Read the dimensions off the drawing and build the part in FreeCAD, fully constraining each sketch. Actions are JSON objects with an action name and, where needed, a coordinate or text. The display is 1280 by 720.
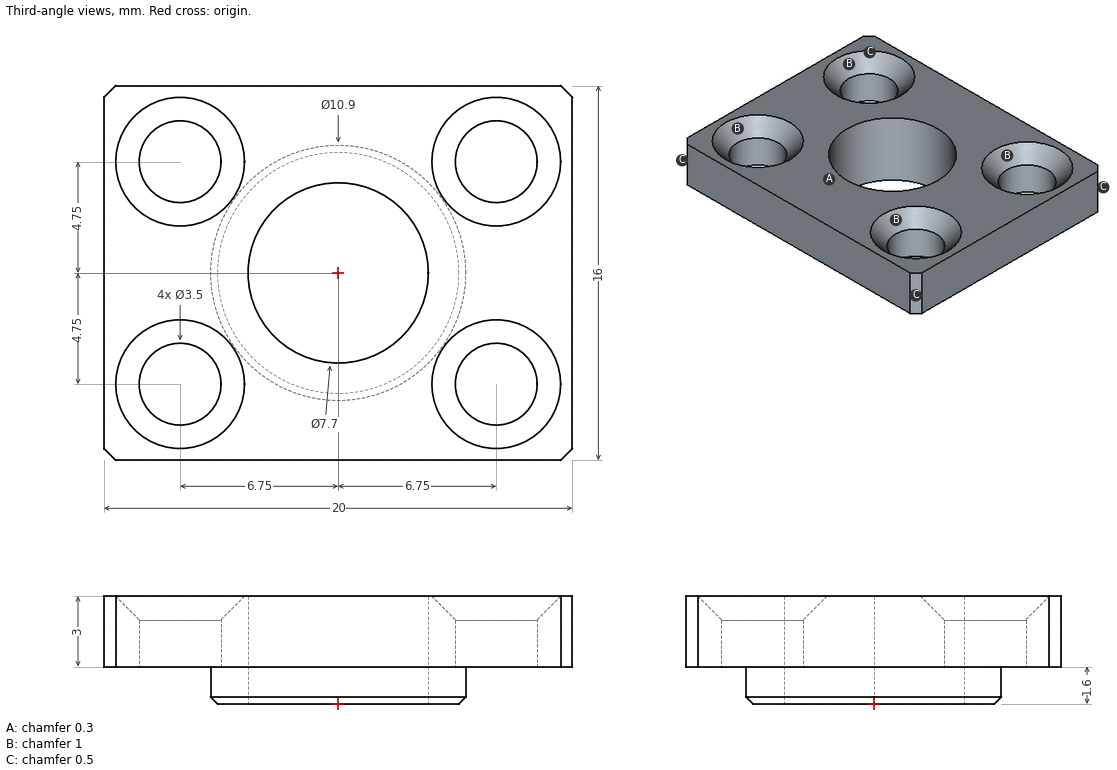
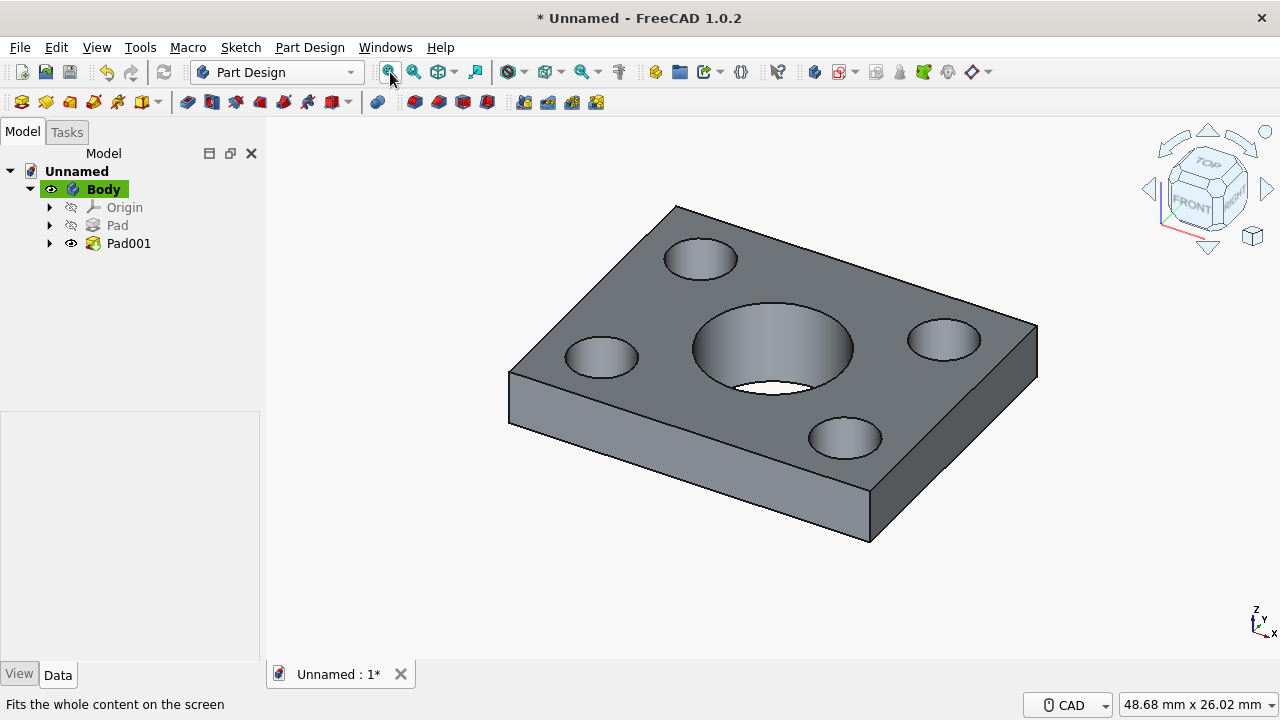
{"action": "key", "text": "0"}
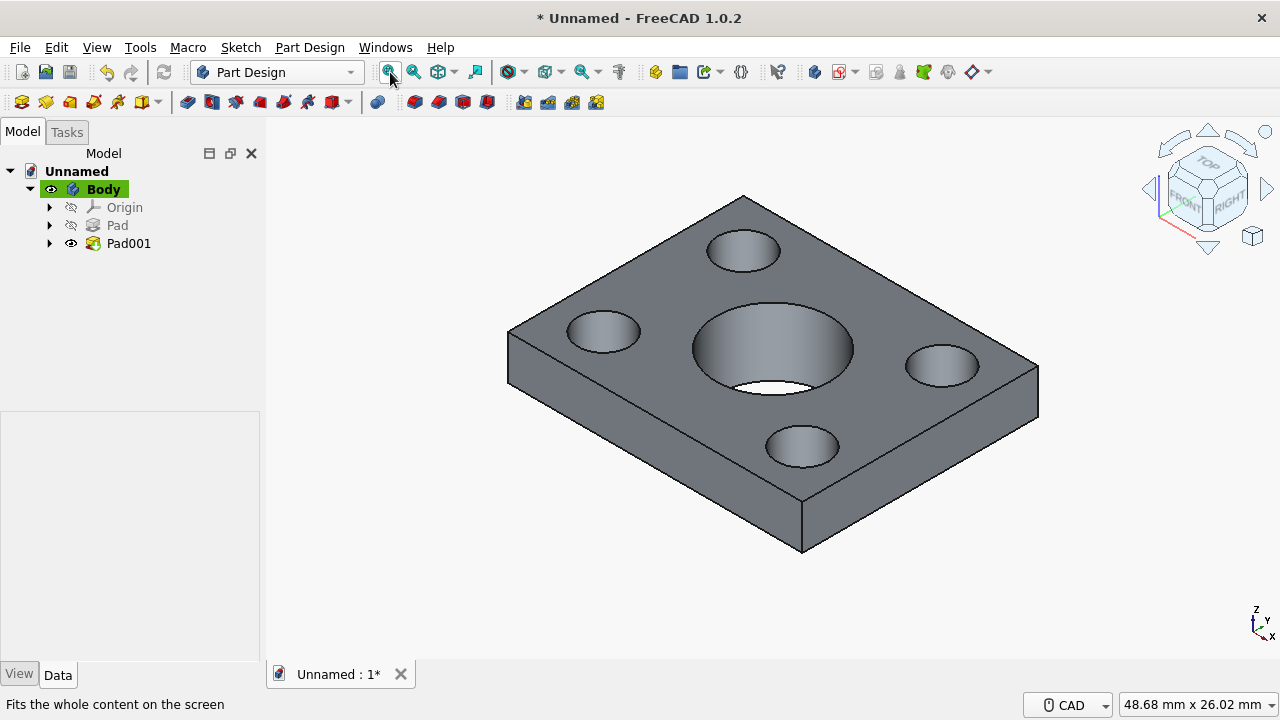
{"action": "key", "text": "2"}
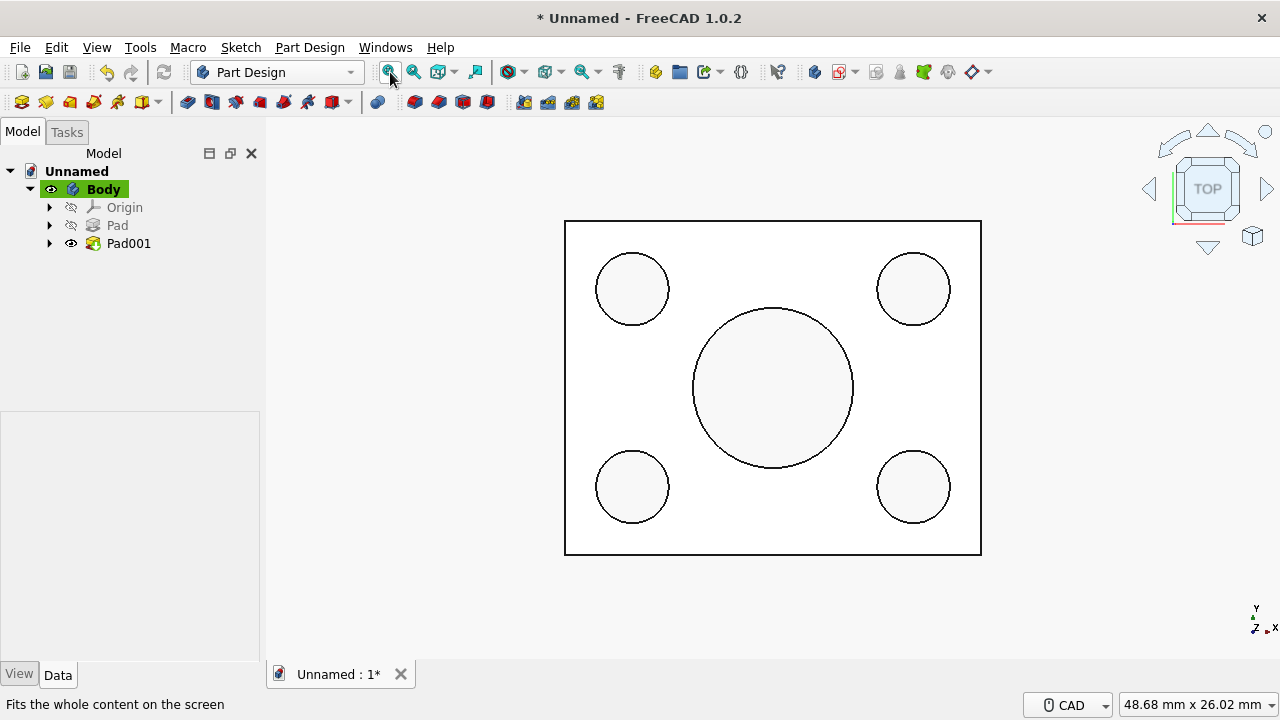
{"action": "key", "text": "1"}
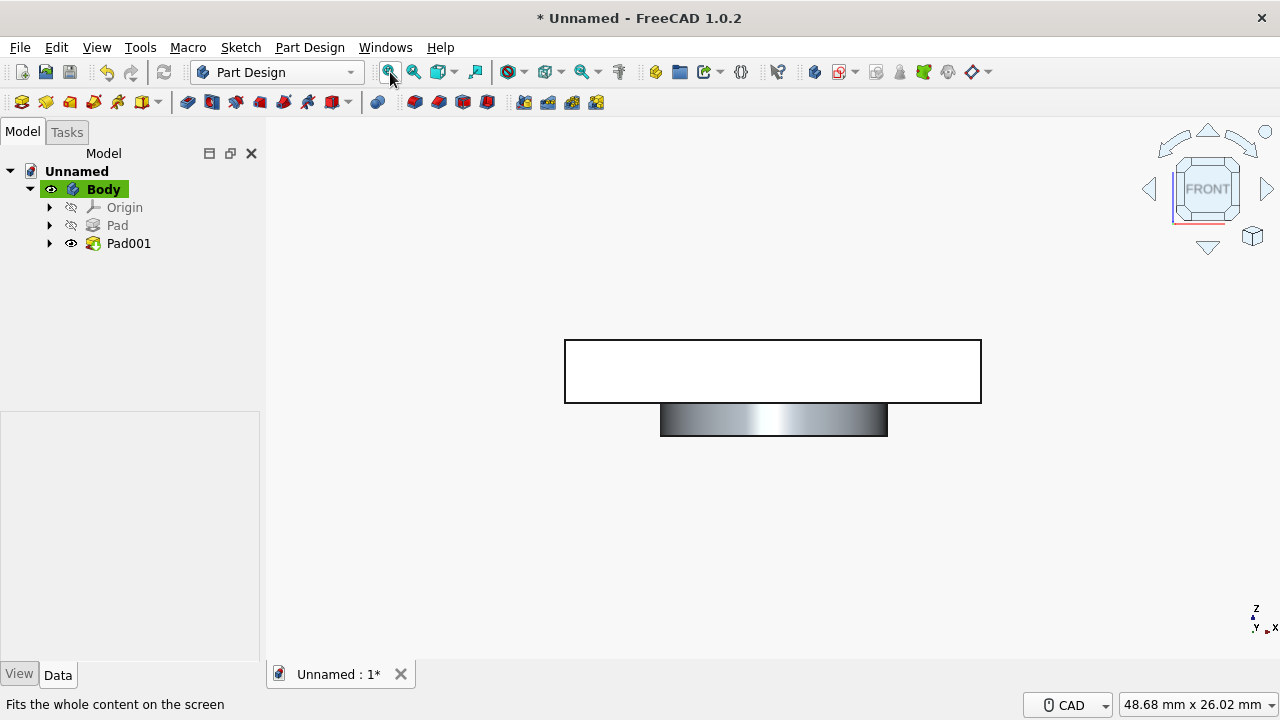
{"action": "key", "text": "v f"}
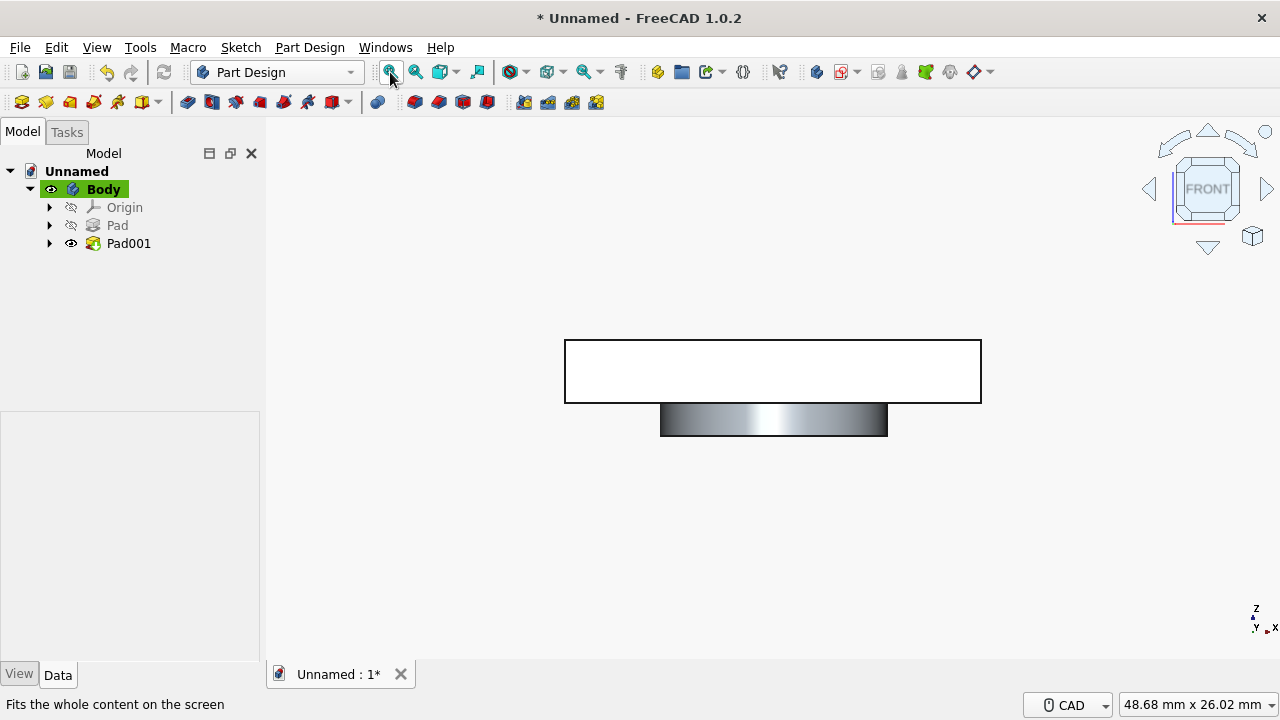
{"action": "left_click", "coordinate": [681, 435]}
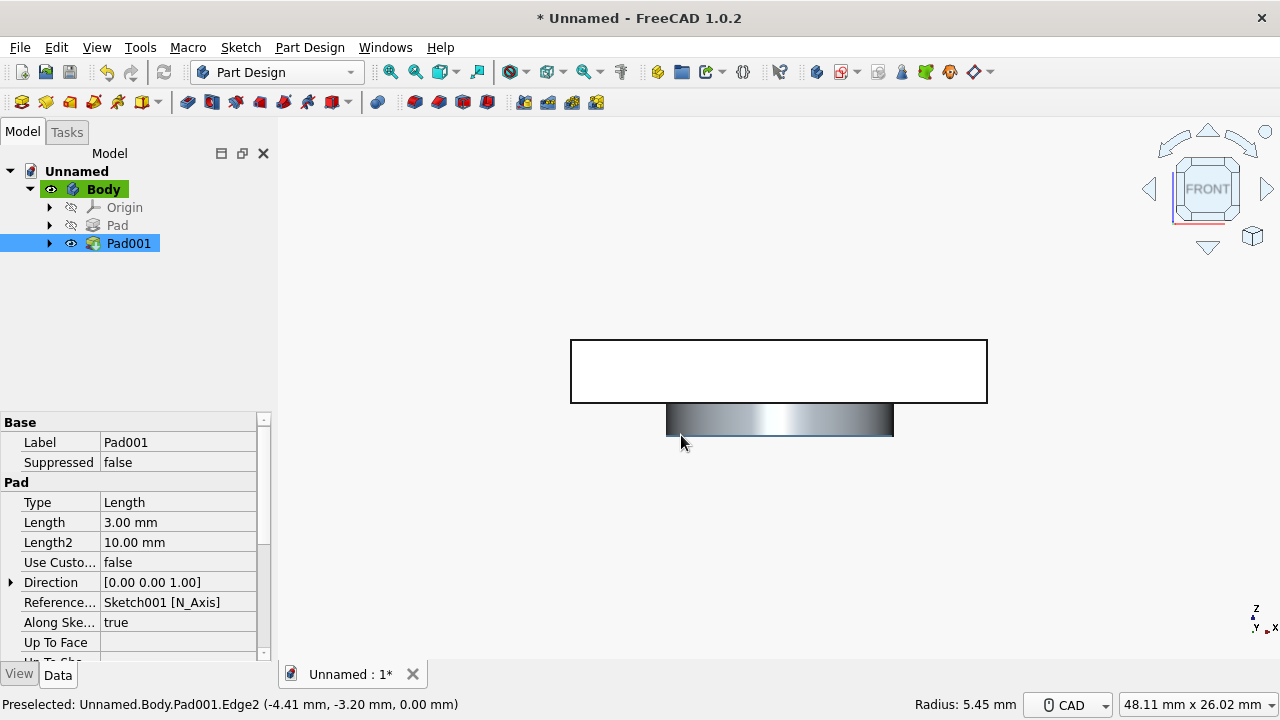
{"action": "left_click", "coordinate": [440, 102]}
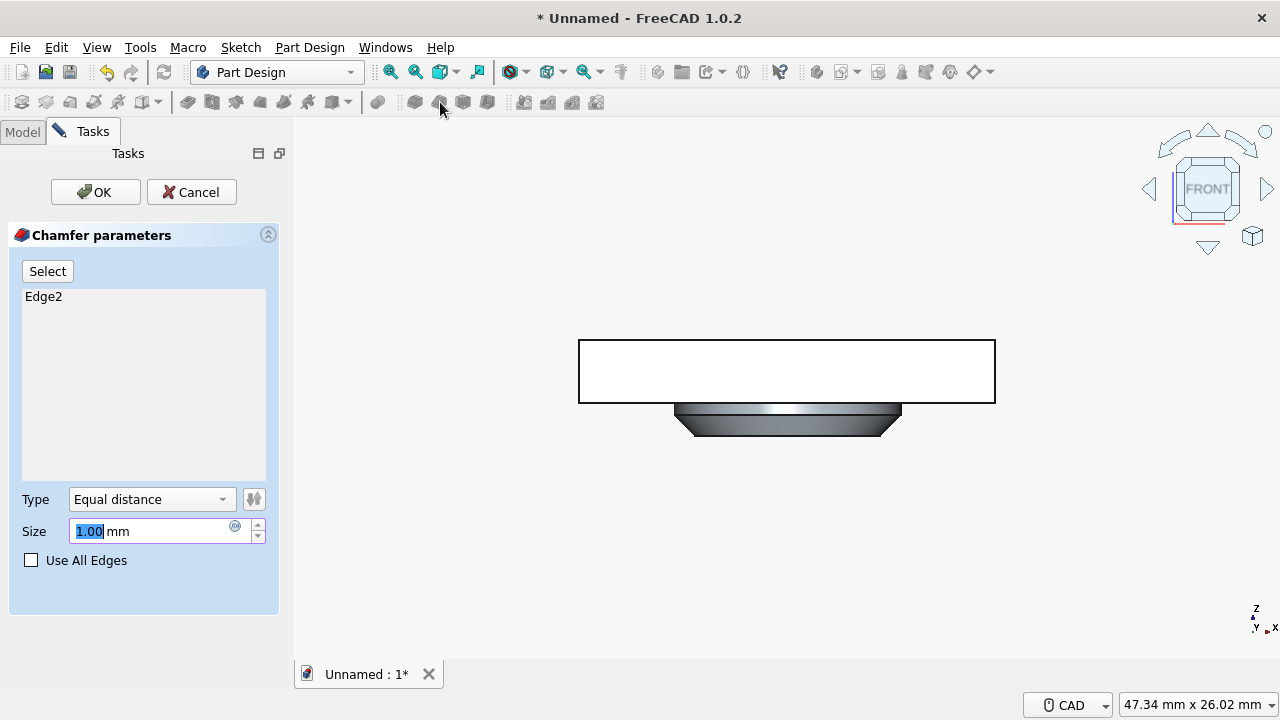
{"action": "type", "text": "0.3"}
{"action": "key", "text": "Tab"}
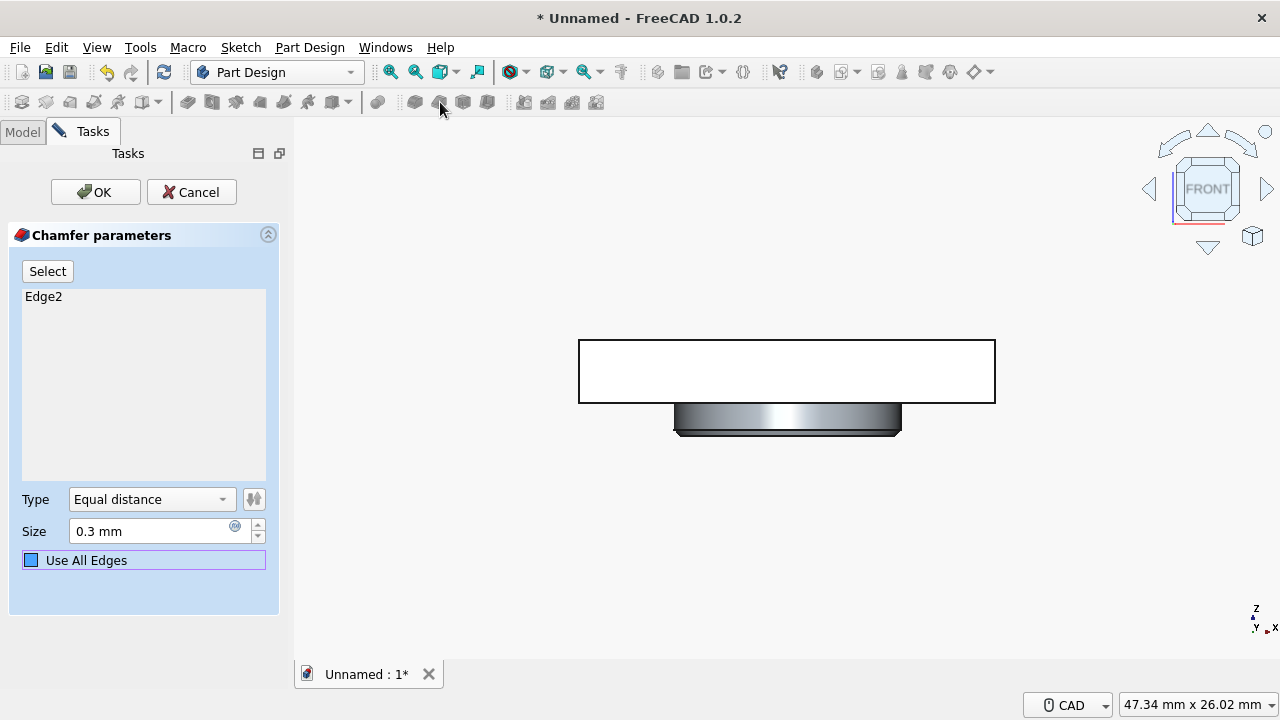
{"action": "left_click", "coordinate": [96, 192]}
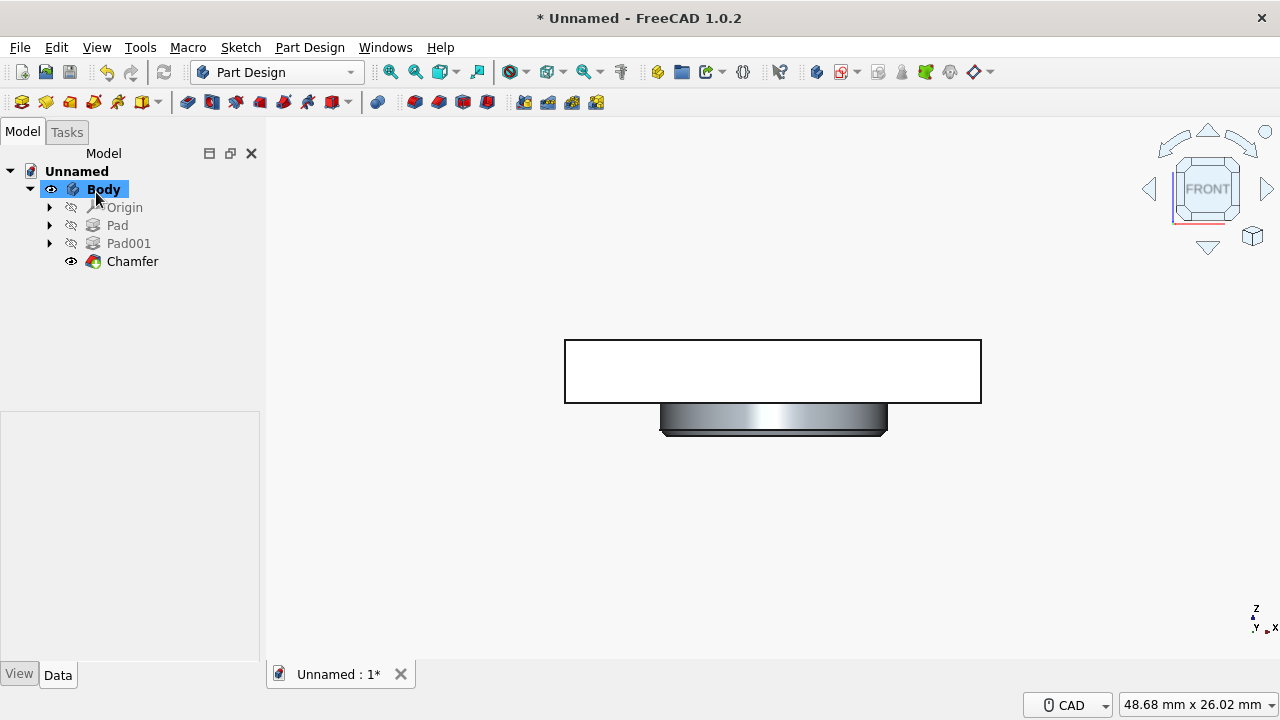
{"action": "left_click", "coordinate": [392, 72]}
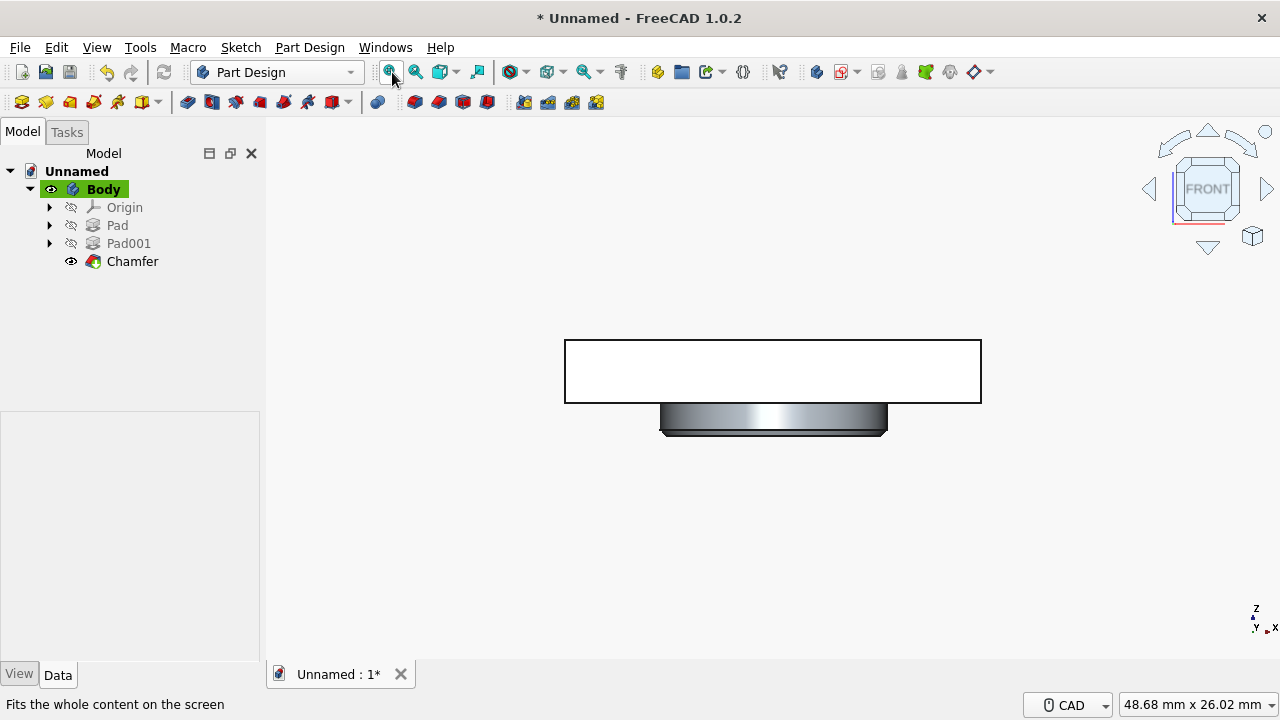
{"action": "key", "text": "0"}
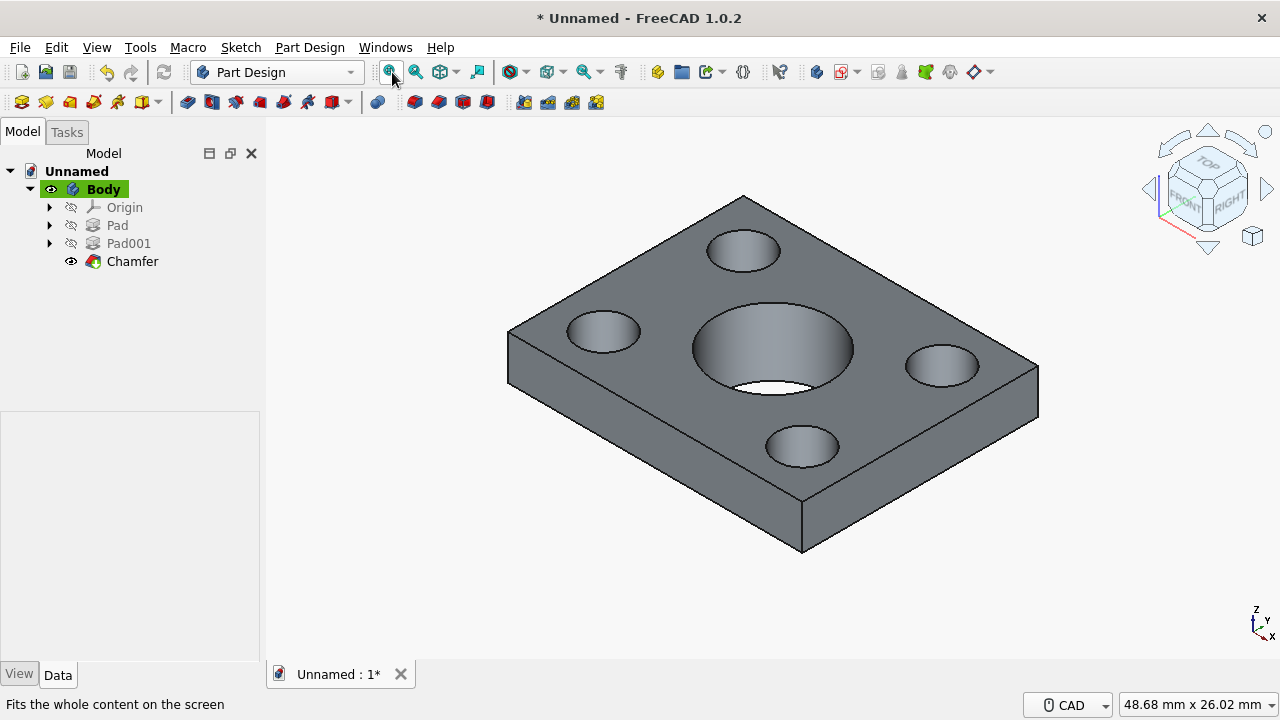
{"action": "left_click", "coordinate": [718, 235]}